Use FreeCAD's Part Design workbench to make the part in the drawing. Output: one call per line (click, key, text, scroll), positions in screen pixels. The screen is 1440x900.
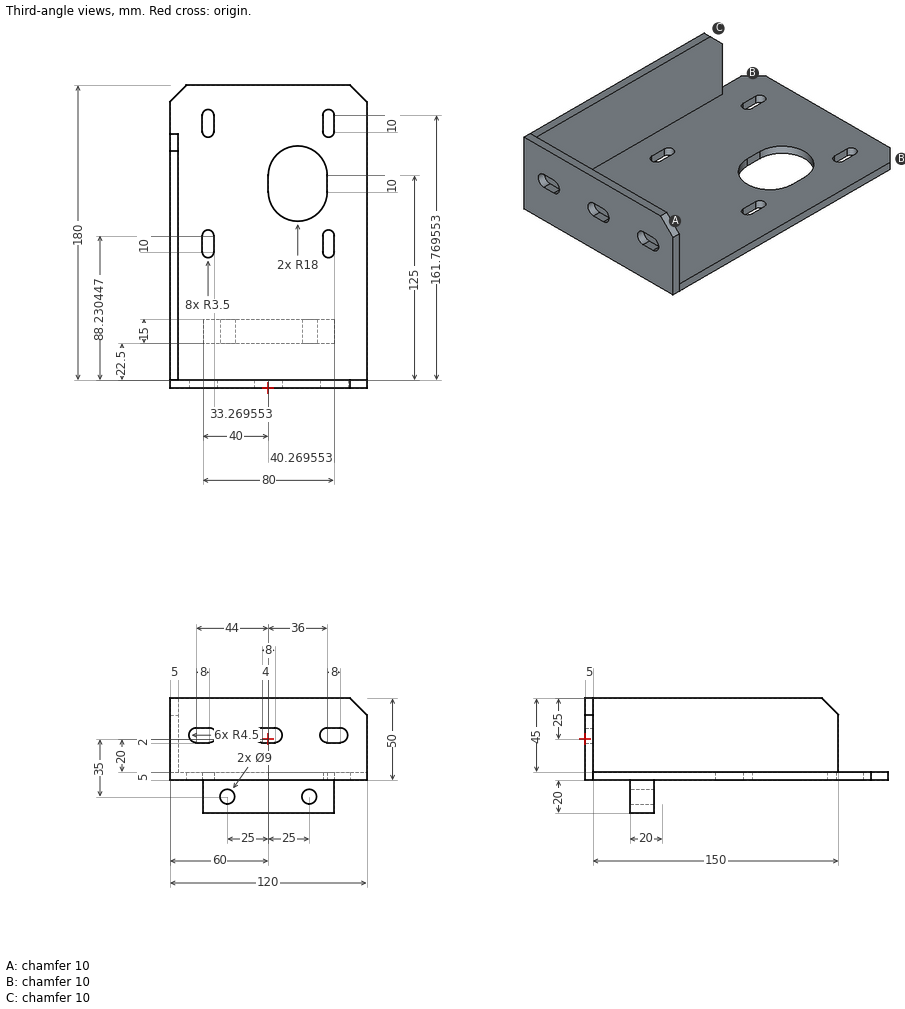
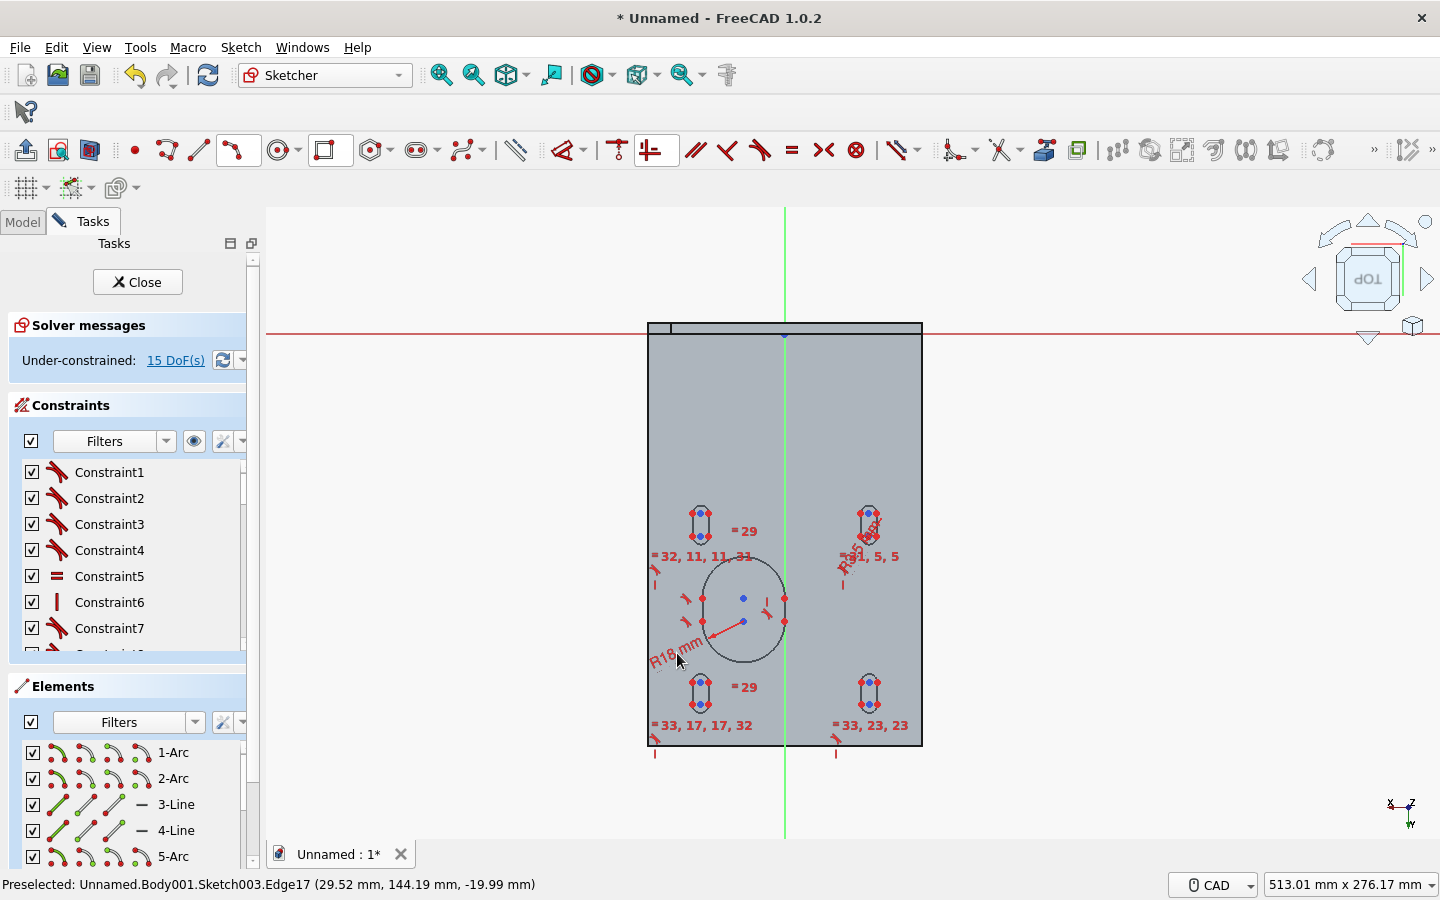
click(785, 621)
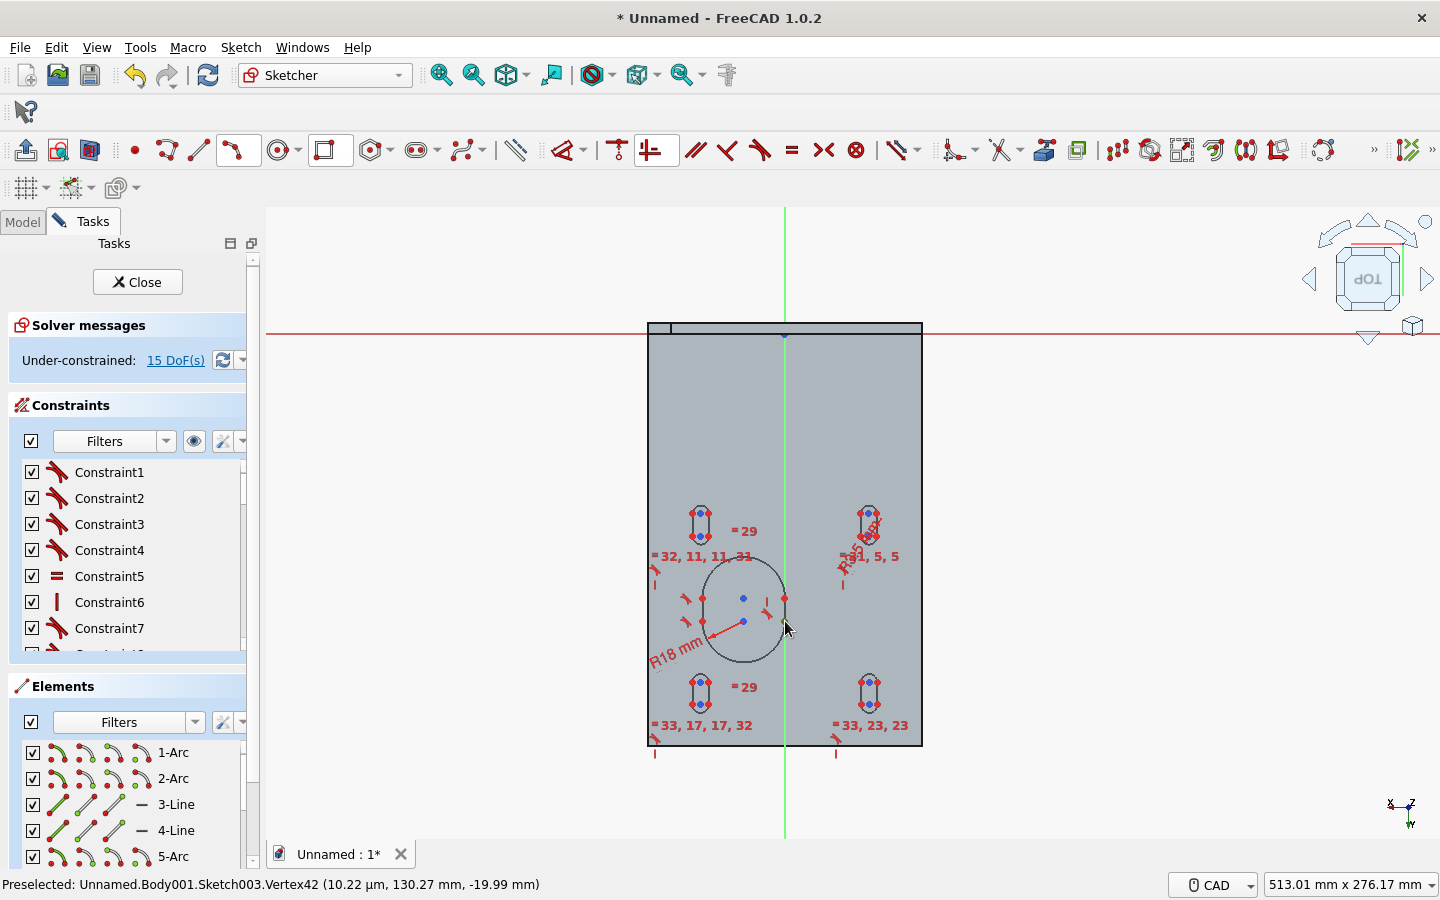
click(785, 770)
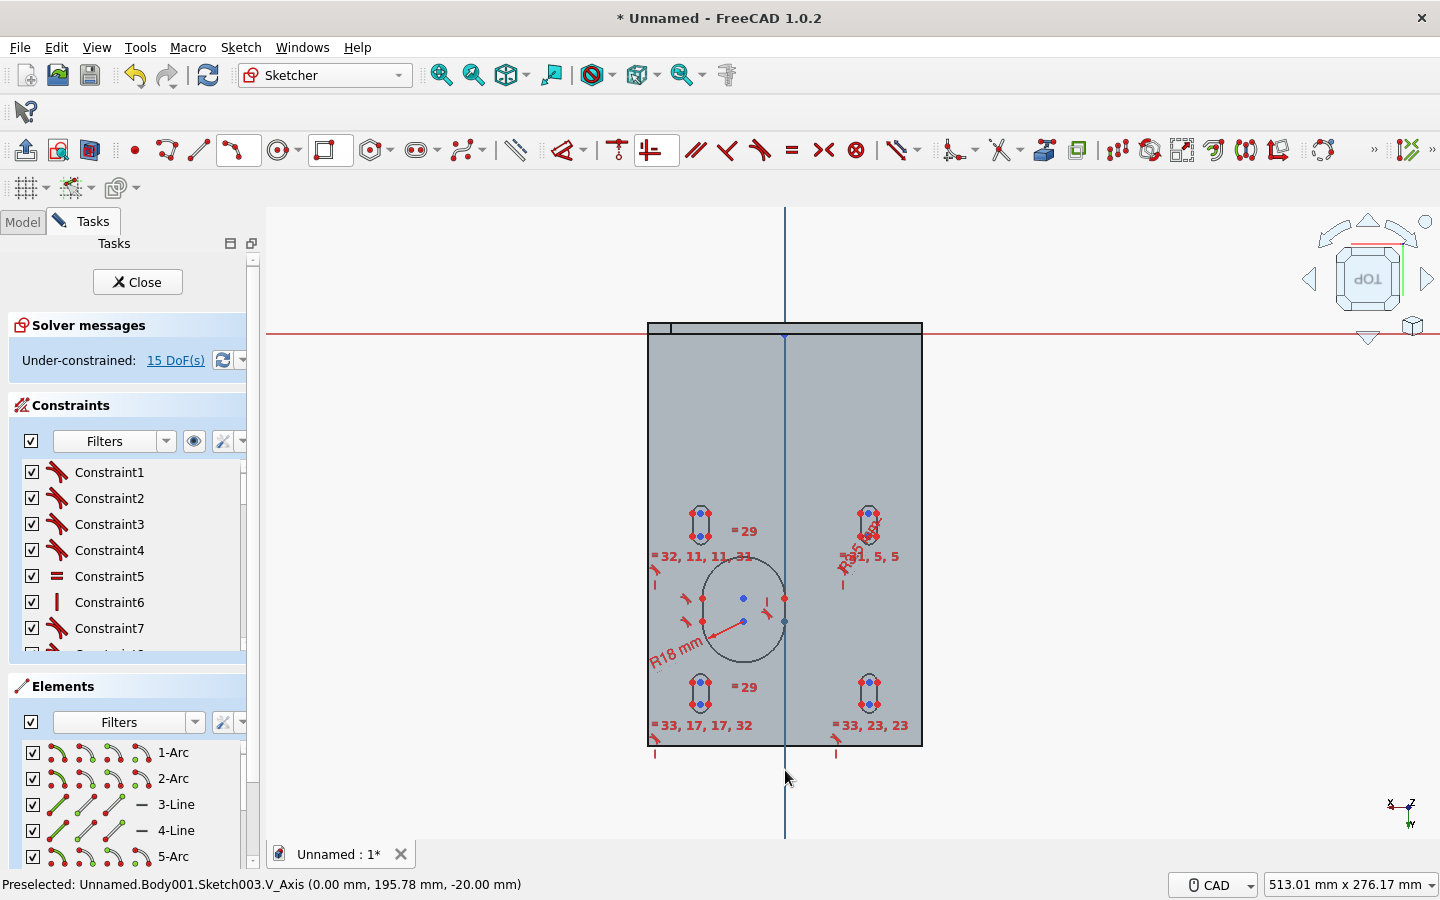
key(c)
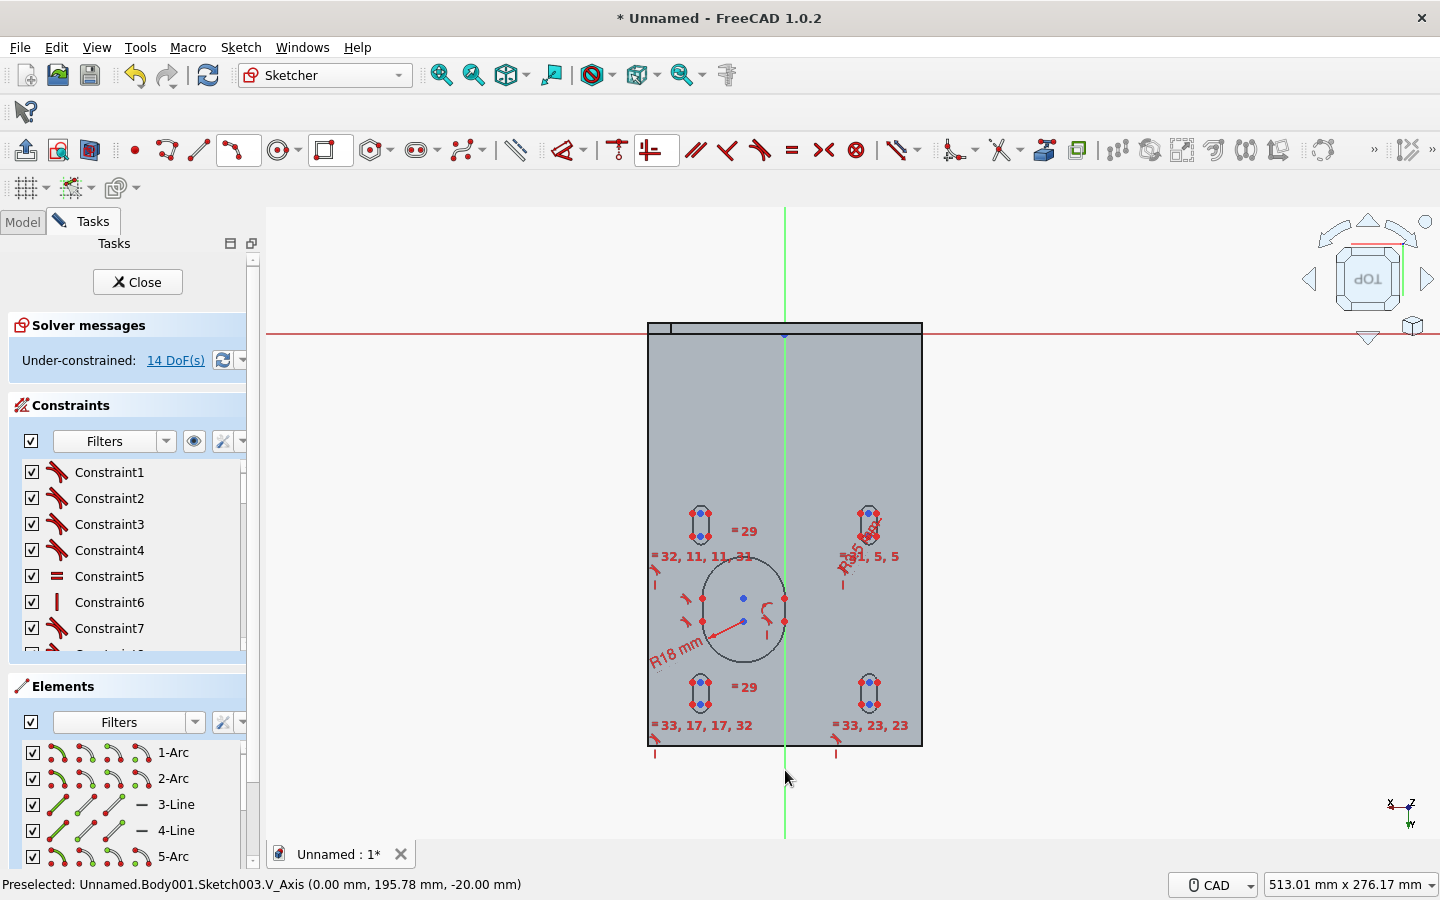
click(562, 150)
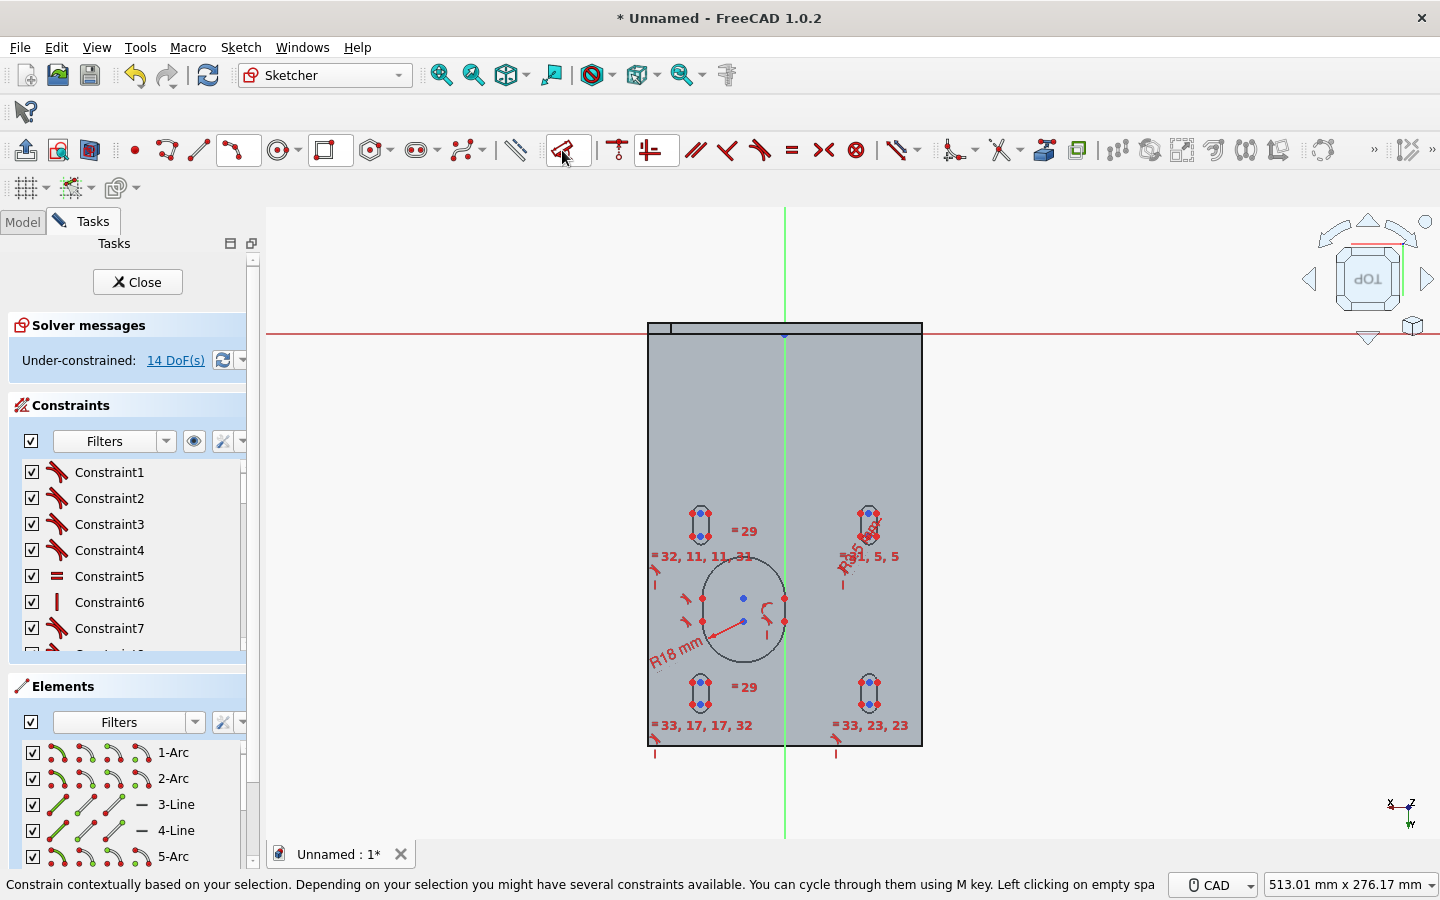
scroll(861, 527, up, 3)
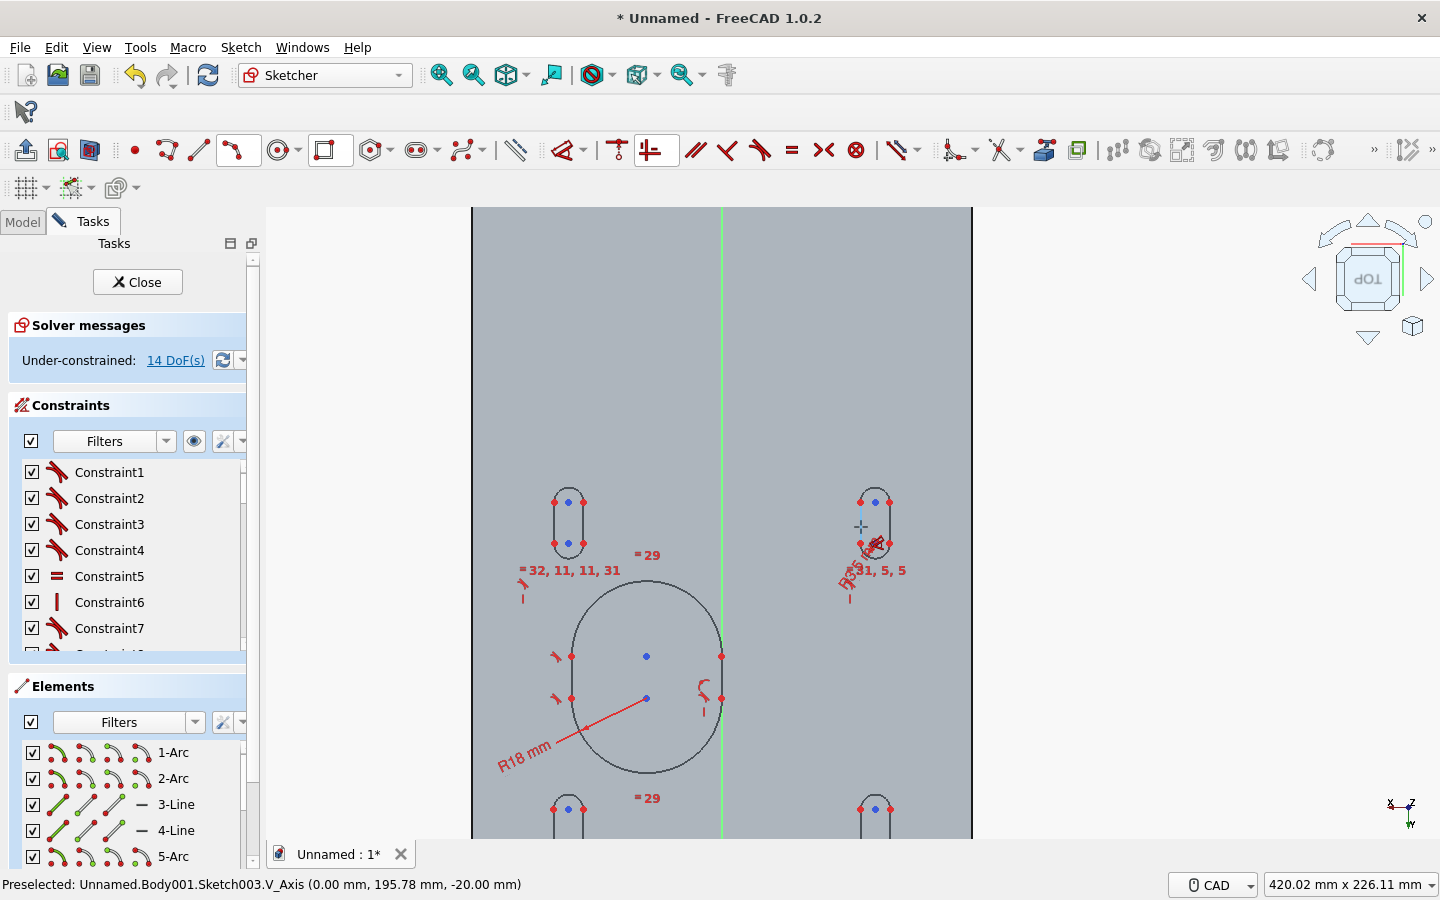
click(861, 527)
click(827, 523)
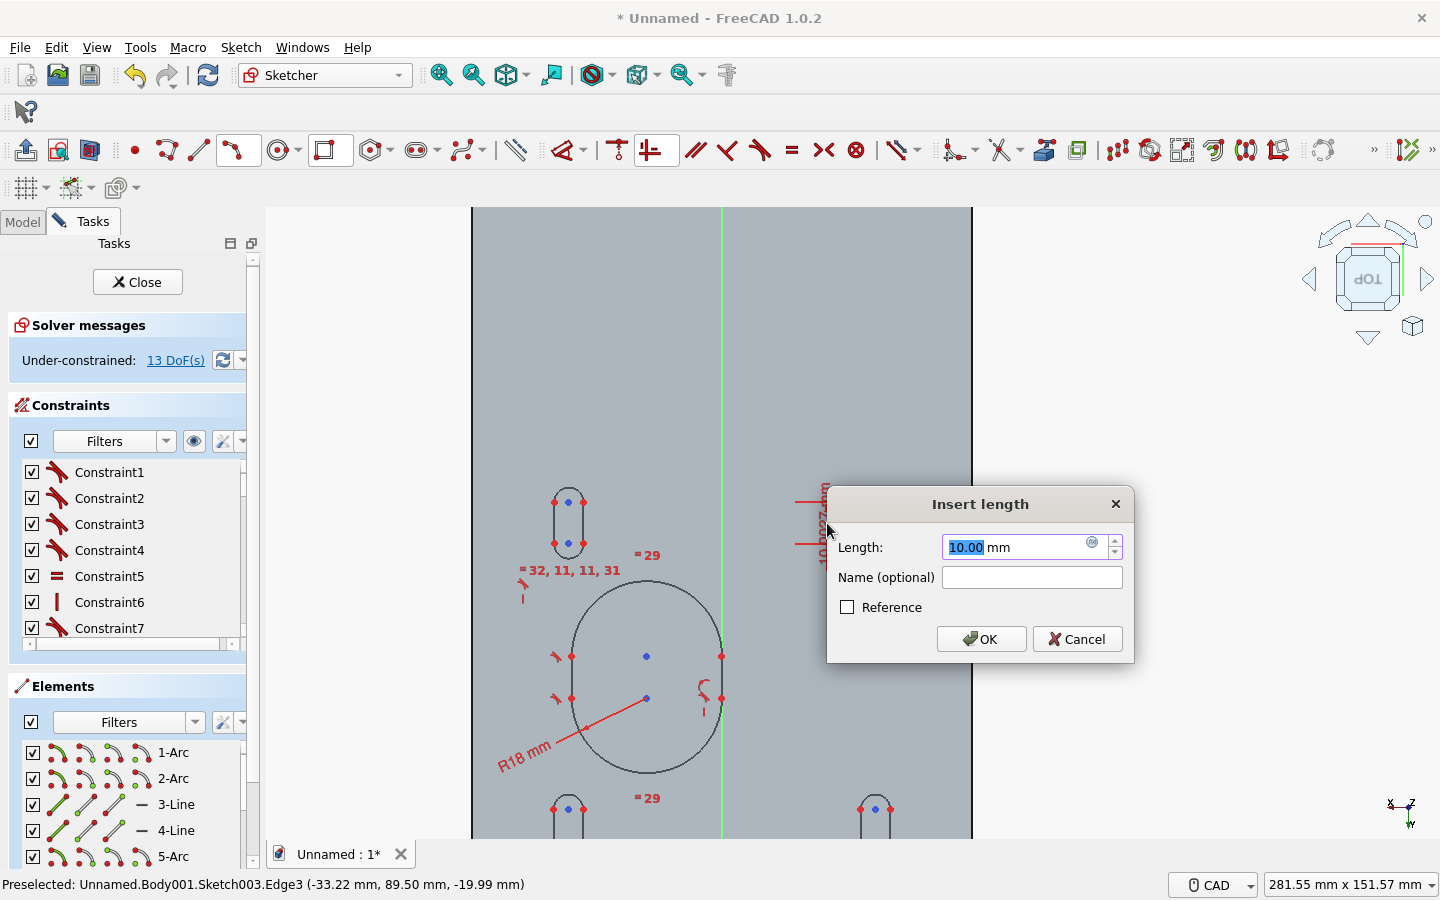
text(10)
key(Return)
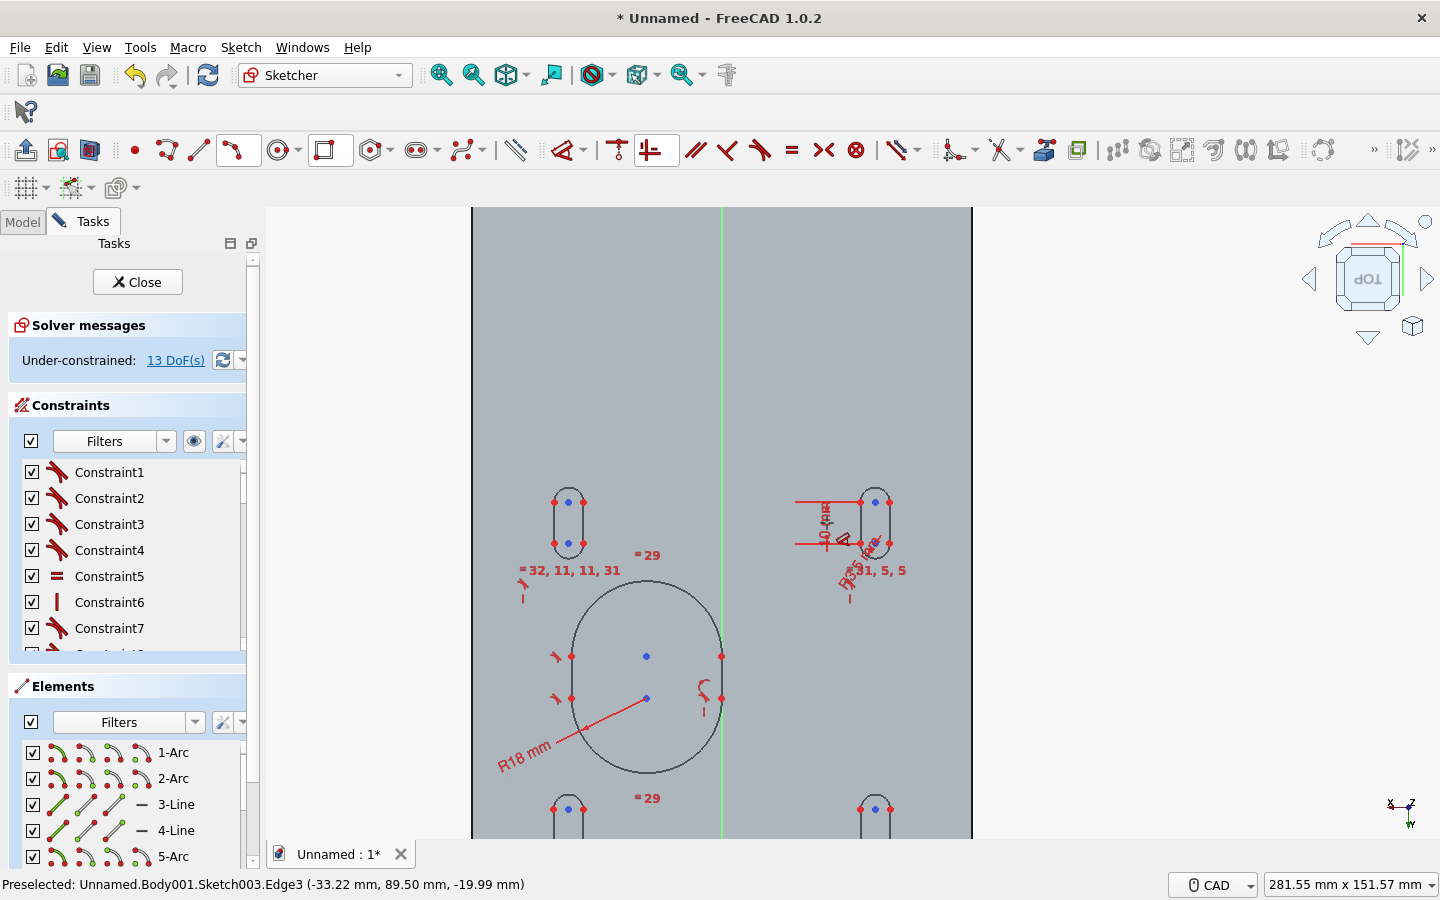
click(554, 531)
click(520, 523)